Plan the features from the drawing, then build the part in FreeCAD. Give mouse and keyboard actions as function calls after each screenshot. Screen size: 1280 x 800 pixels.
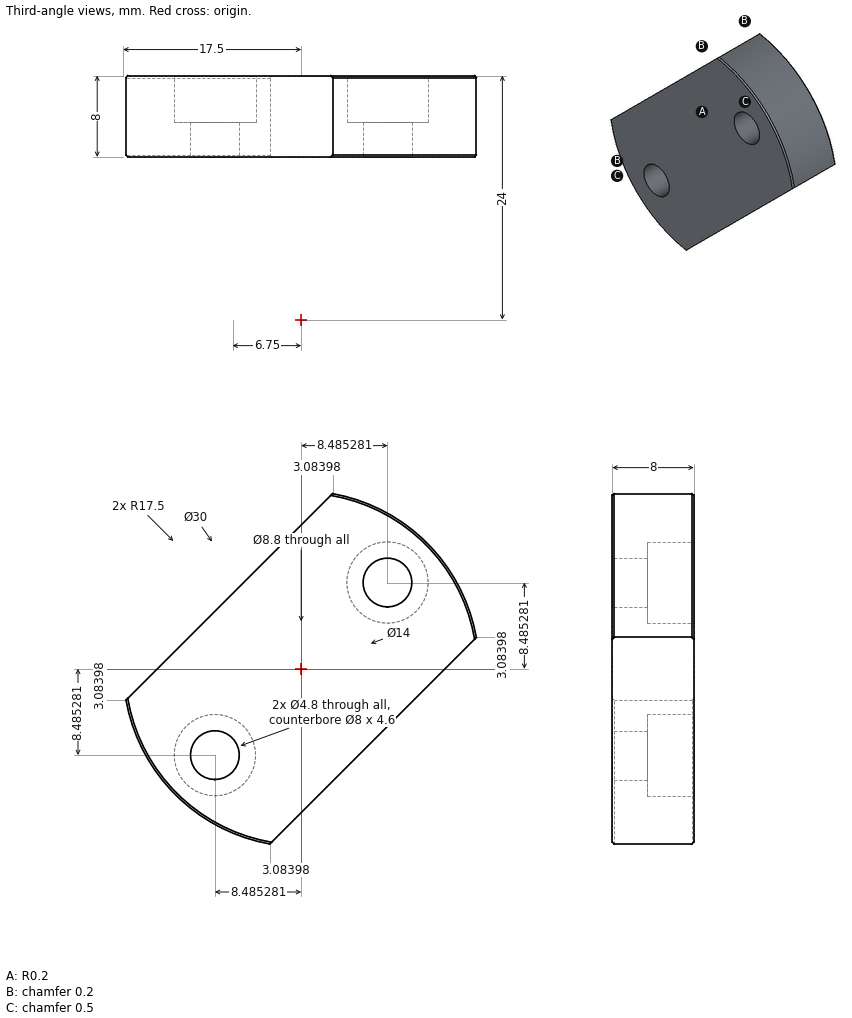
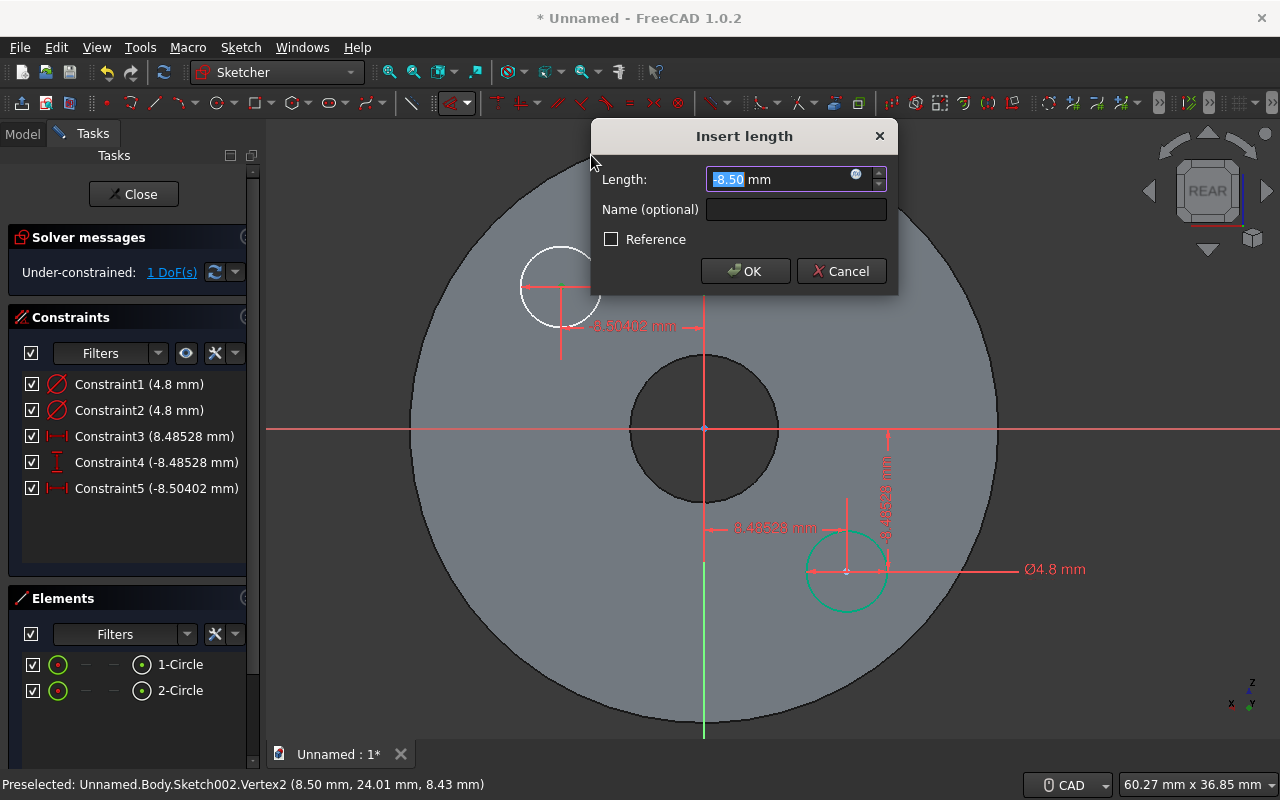
text(-8.485281)
key(Return)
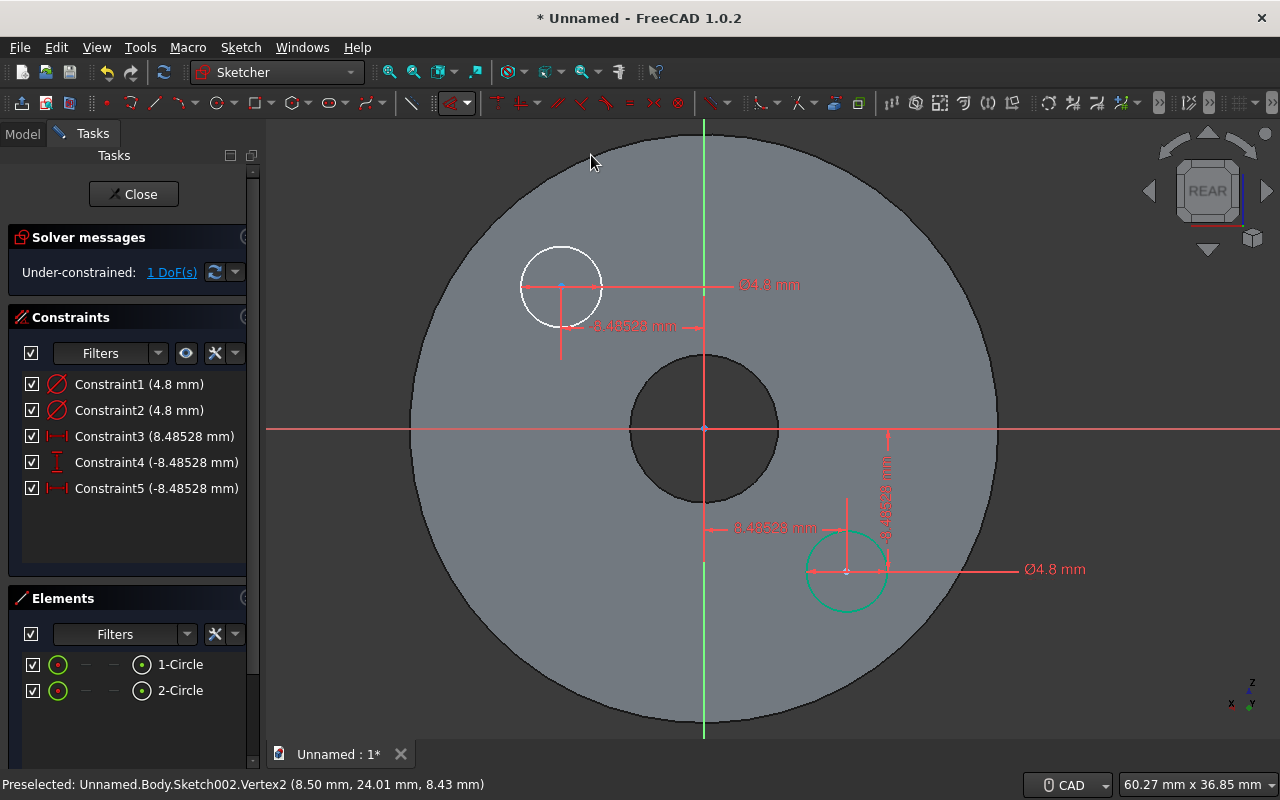
click(561, 287)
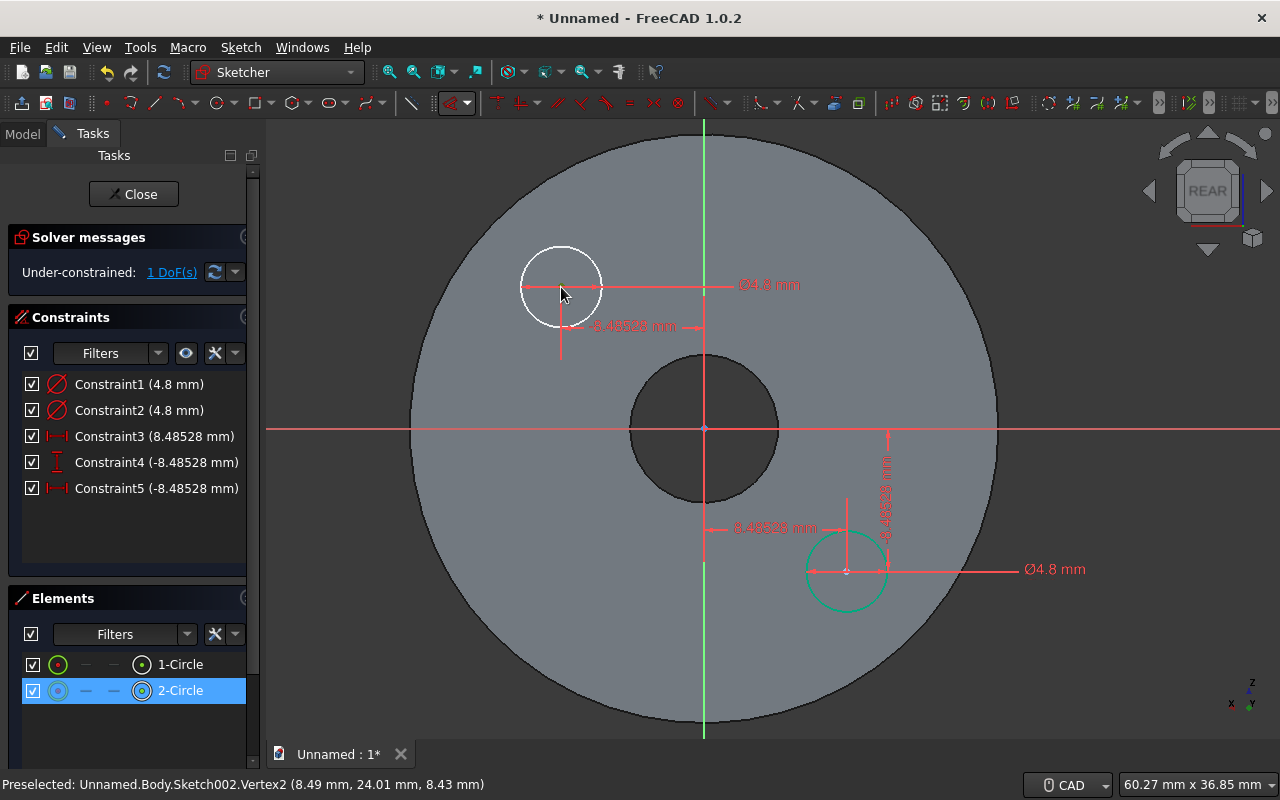
click(470, 104)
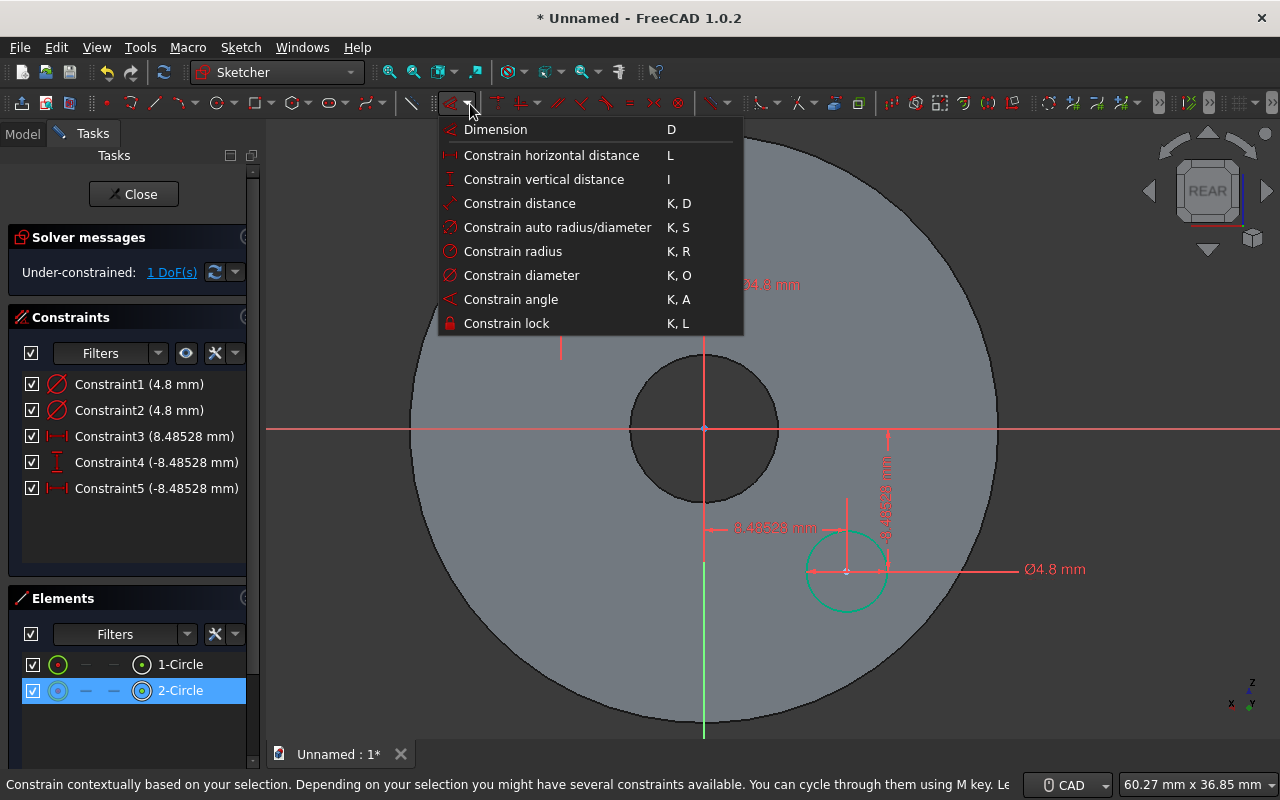
click(591, 179)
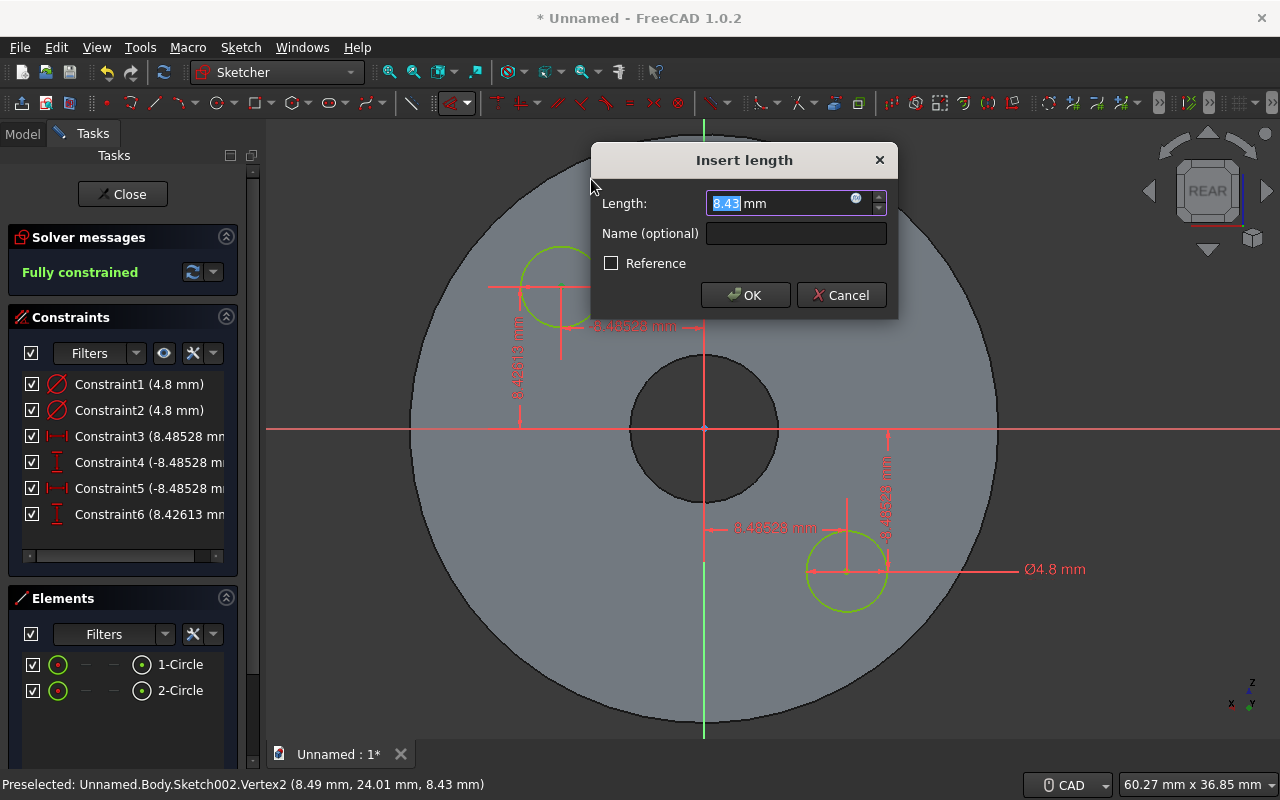
text(8.485281)
key(Return)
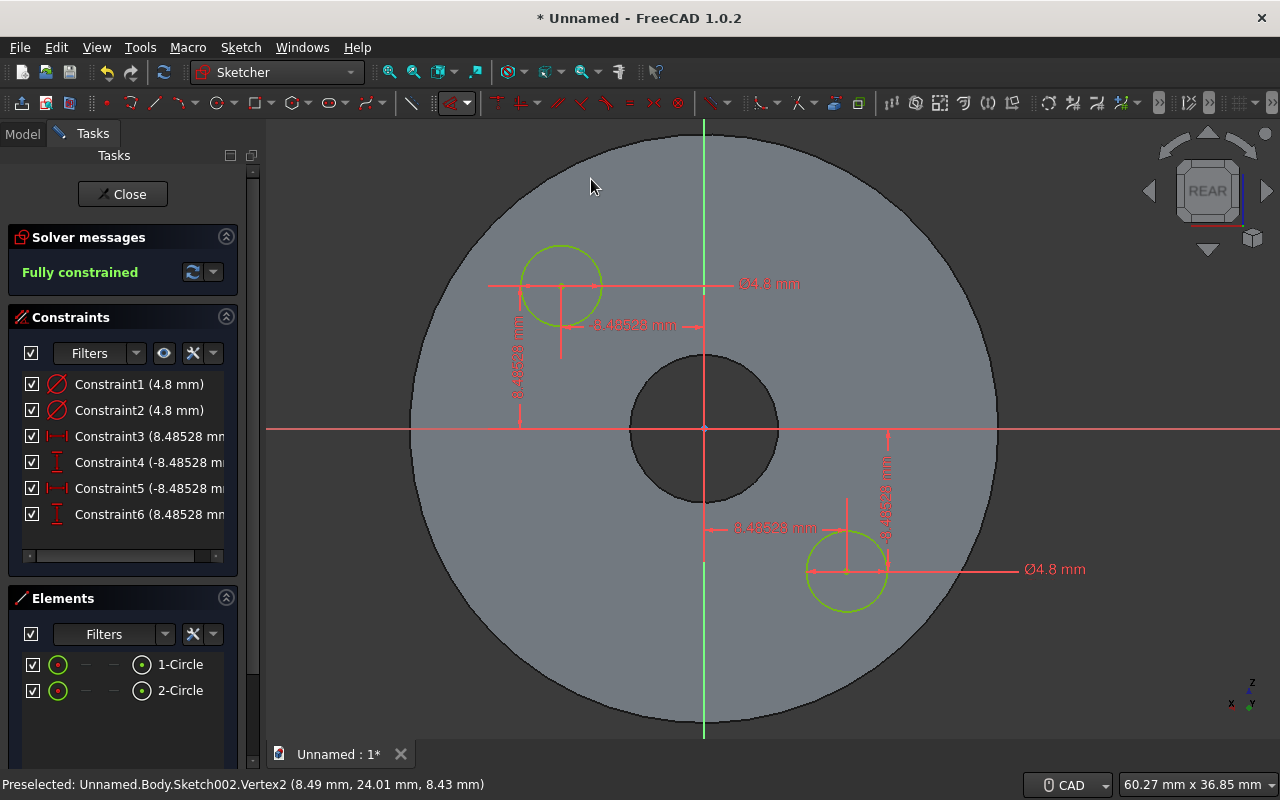
click(123, 194)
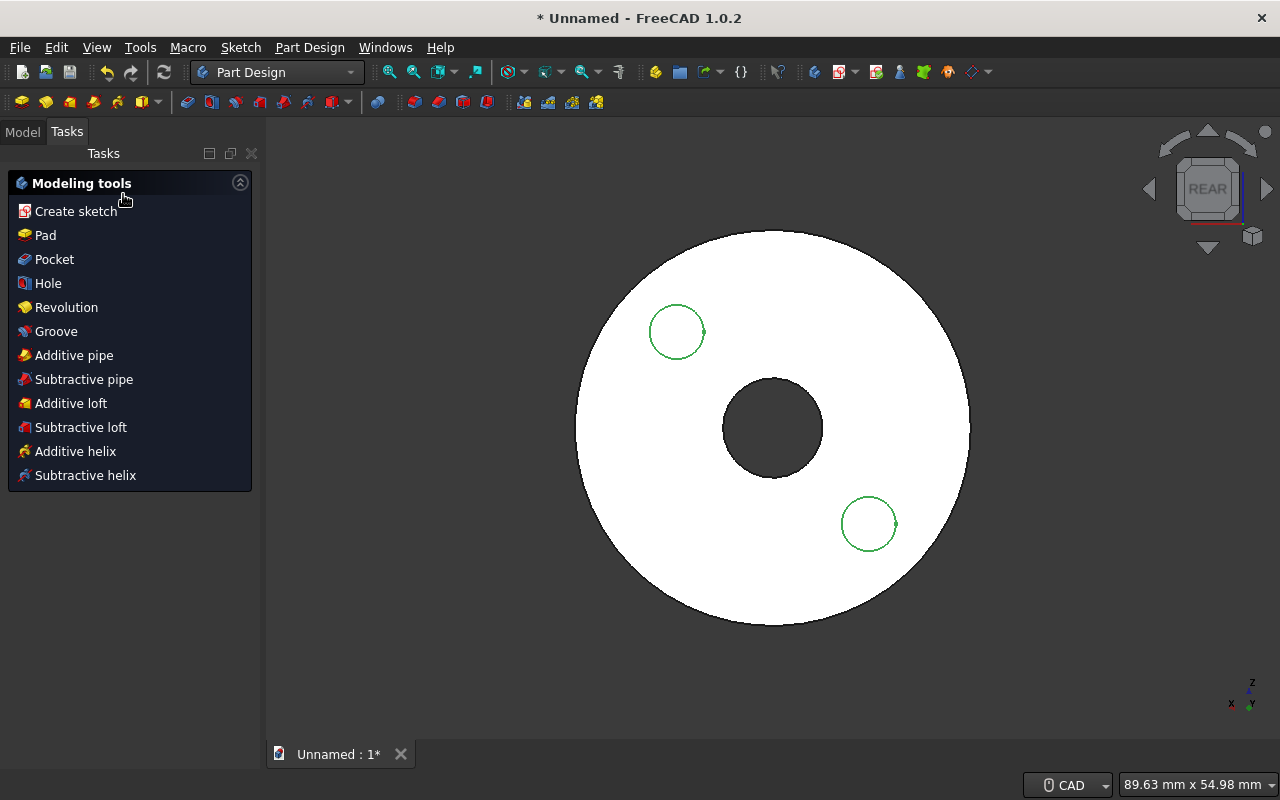
click(212, 102)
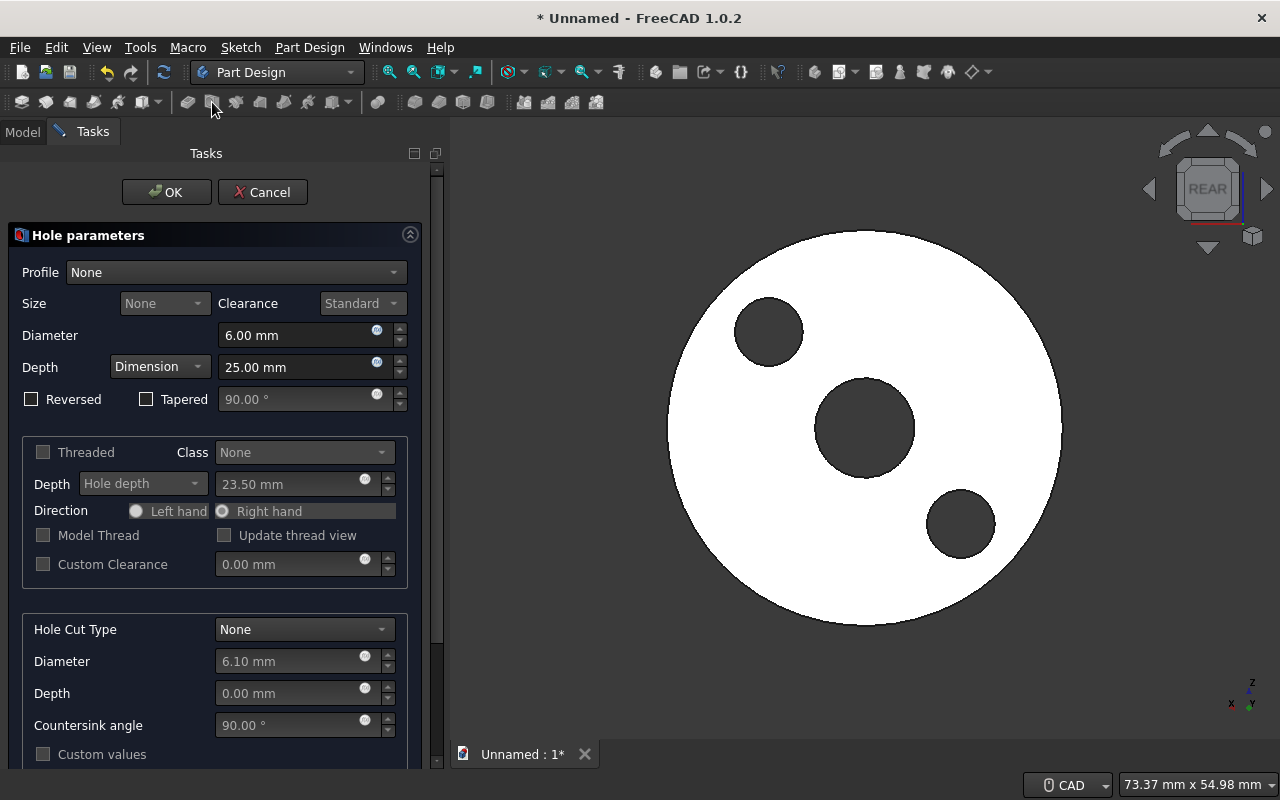
triple_click(305, 335)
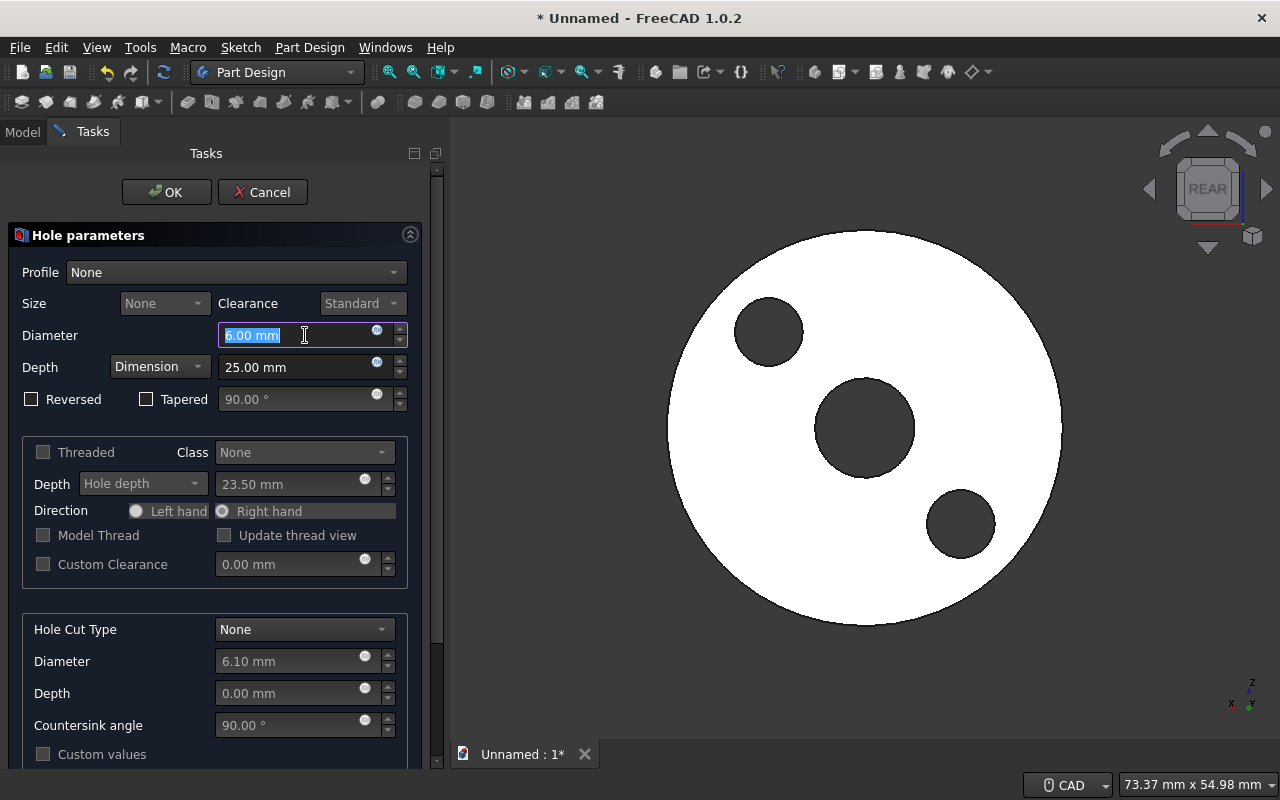
text(4.8)
key(Tab)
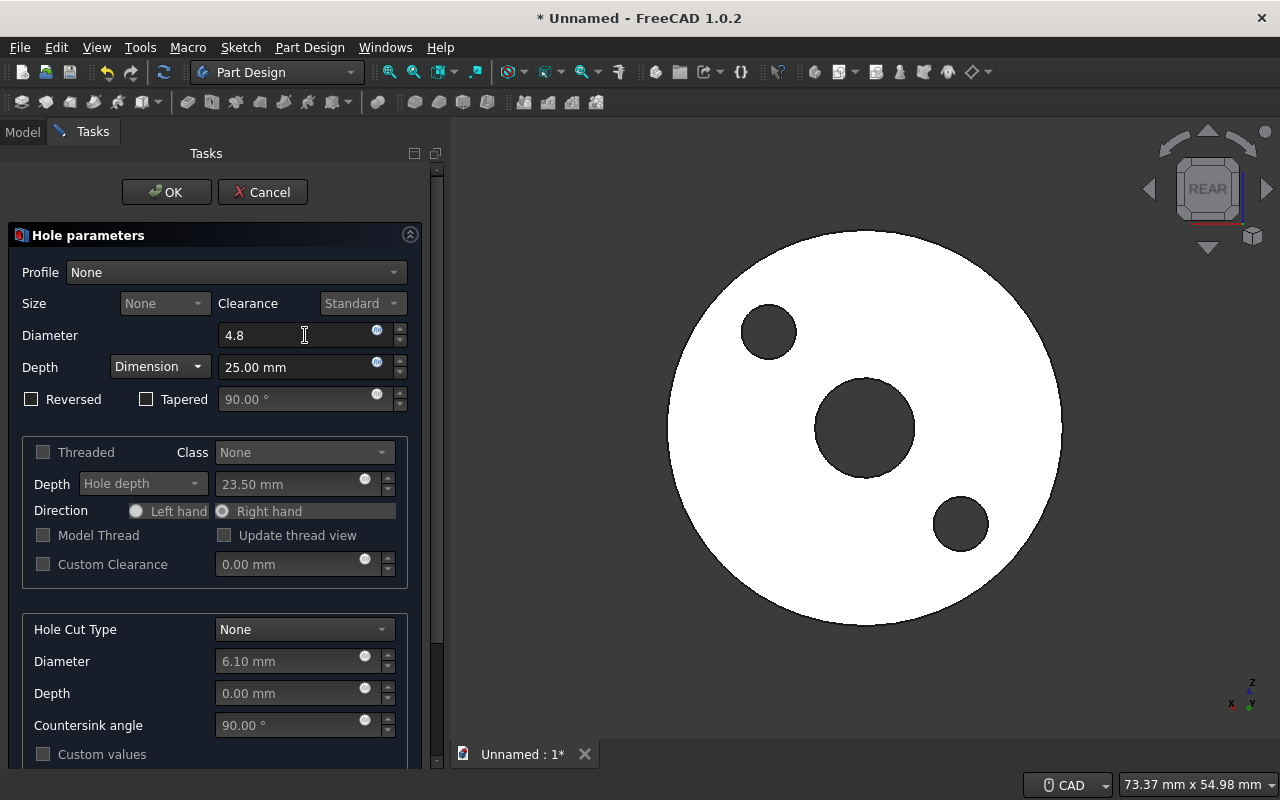
click(161, 366)